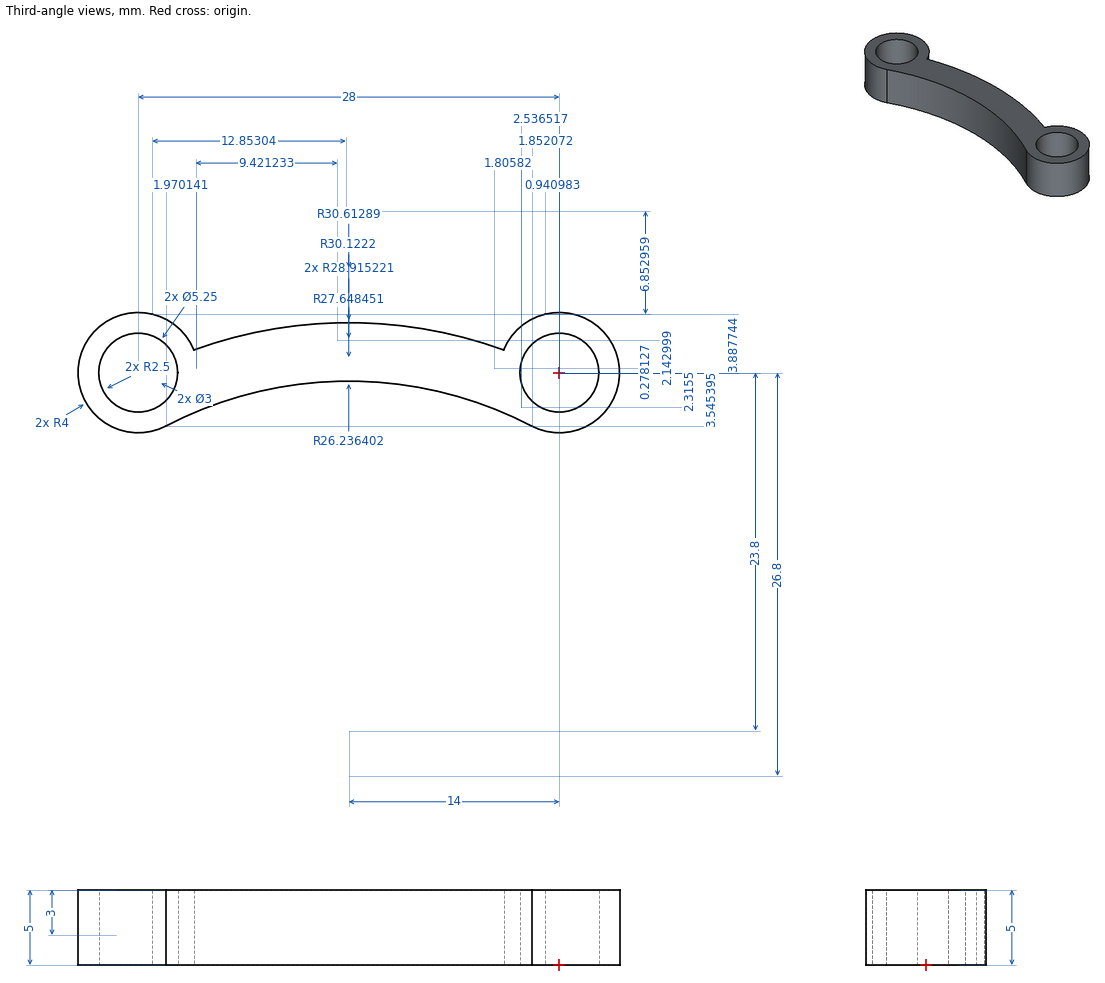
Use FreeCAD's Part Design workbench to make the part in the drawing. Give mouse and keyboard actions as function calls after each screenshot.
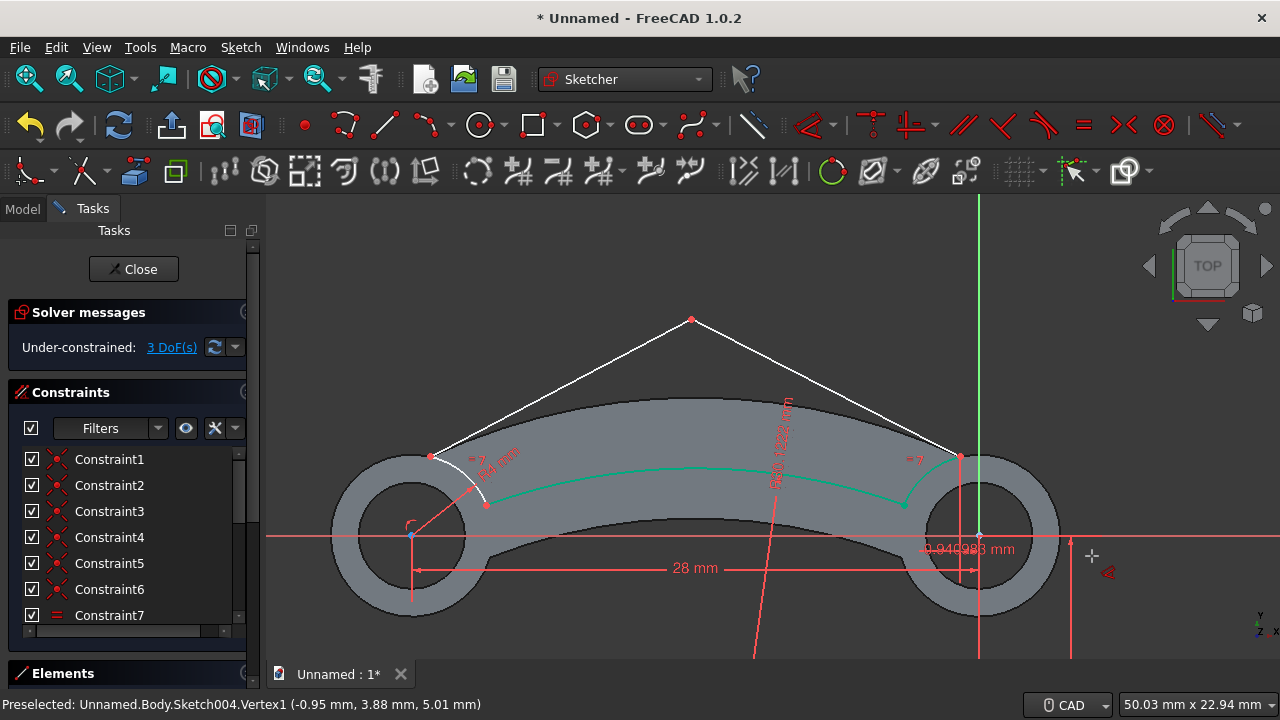
click(431, 457)
click(397, 496)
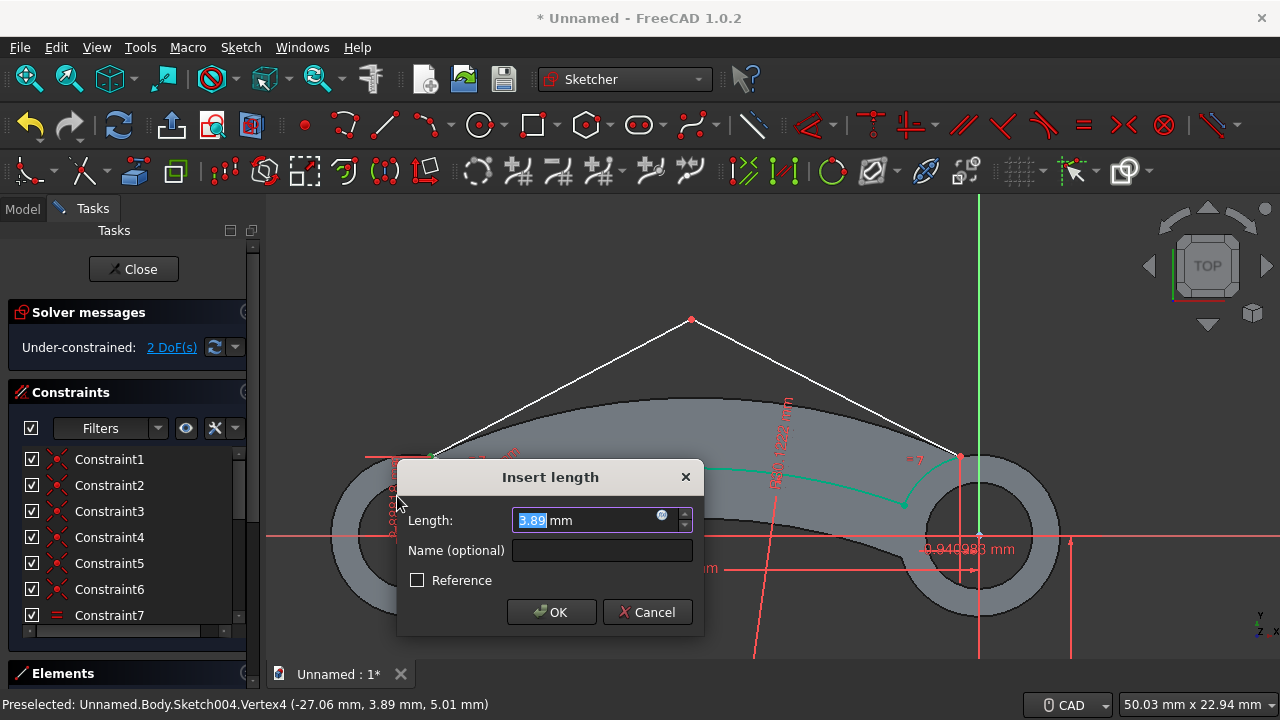
text(3.887744)
key(Return)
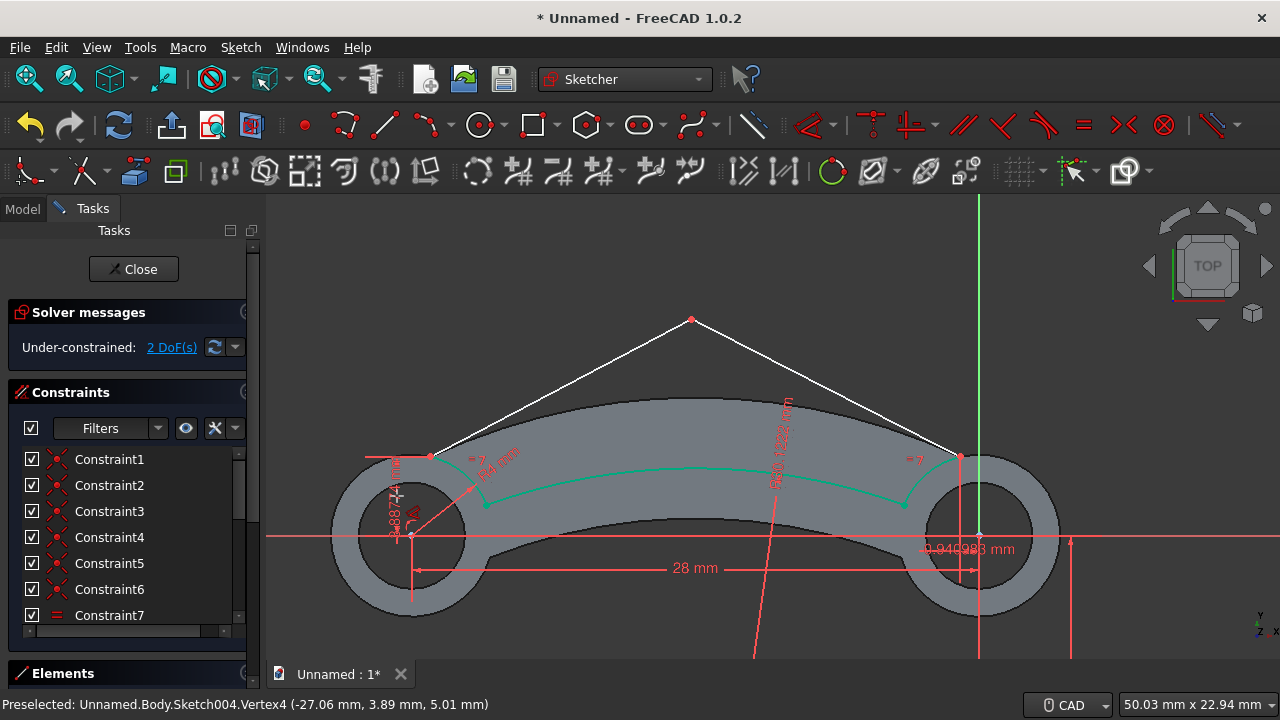
click(880, 416)
click(994, 388)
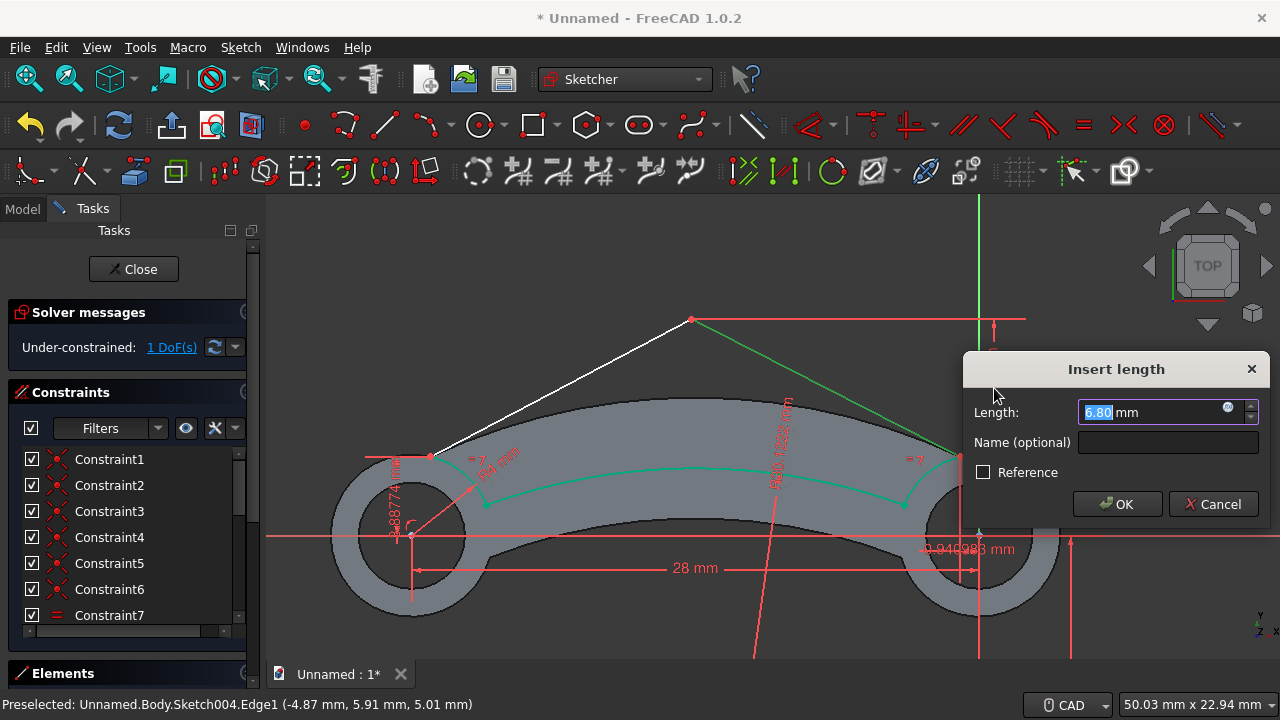
text(6.852959)
key(Return)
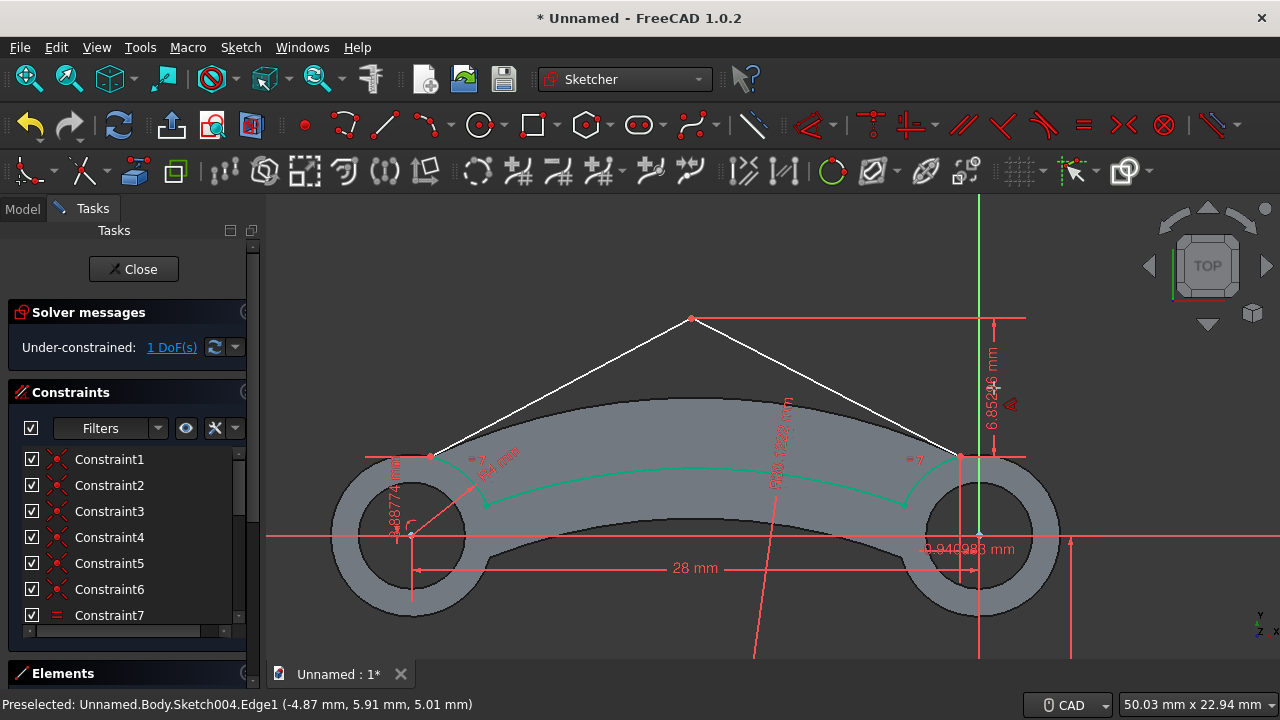
click(614, 360)
click(561, 284)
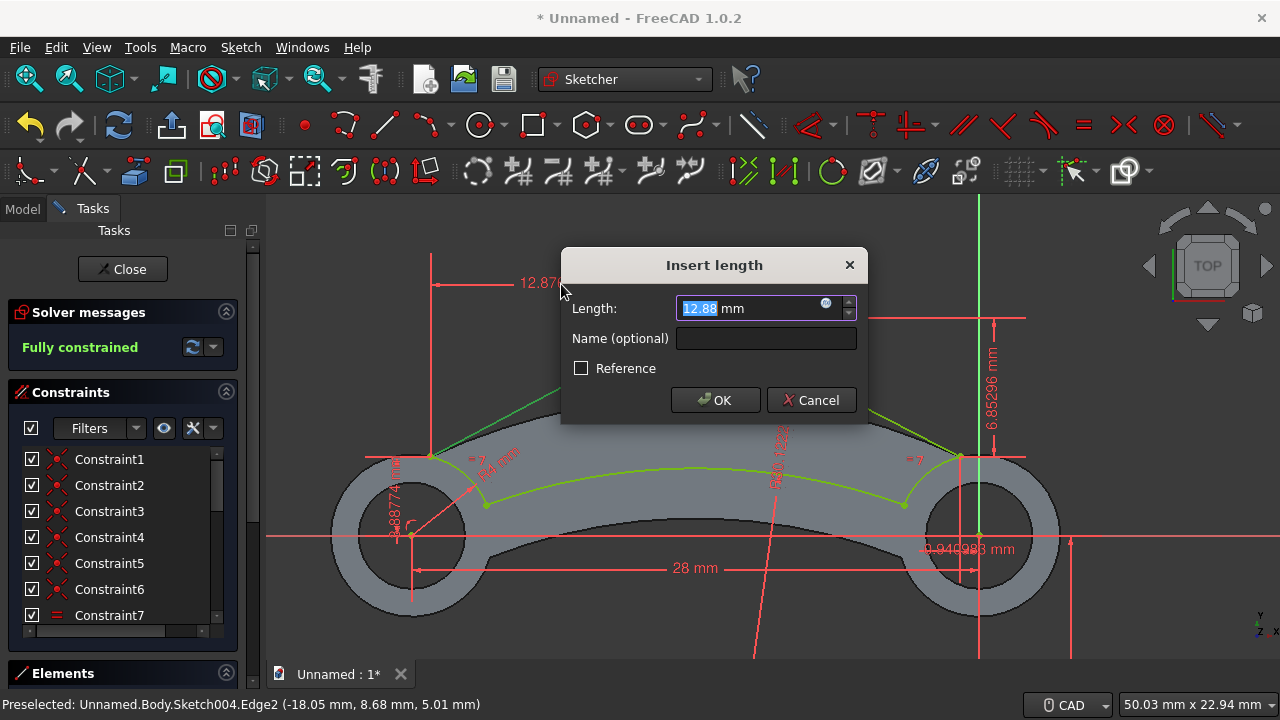
text(12.85304)
key(Return)
key(Escape)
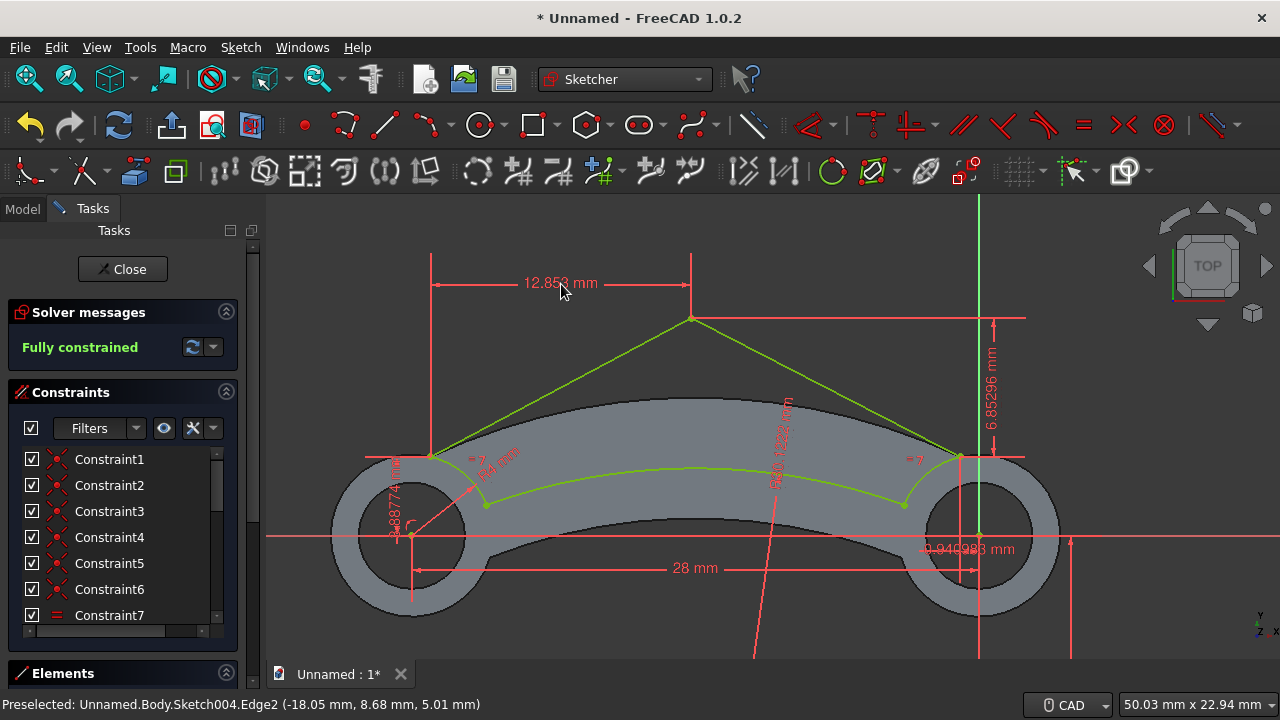
click(123, 269)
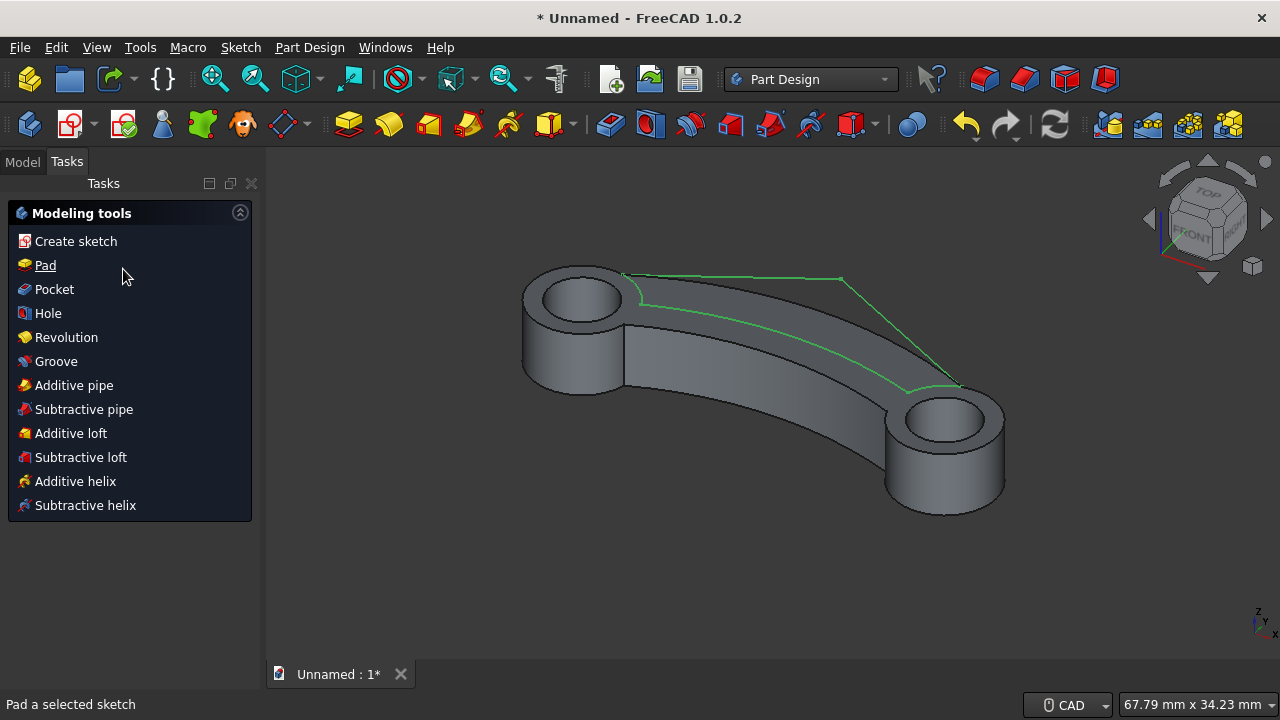
click(612, 124)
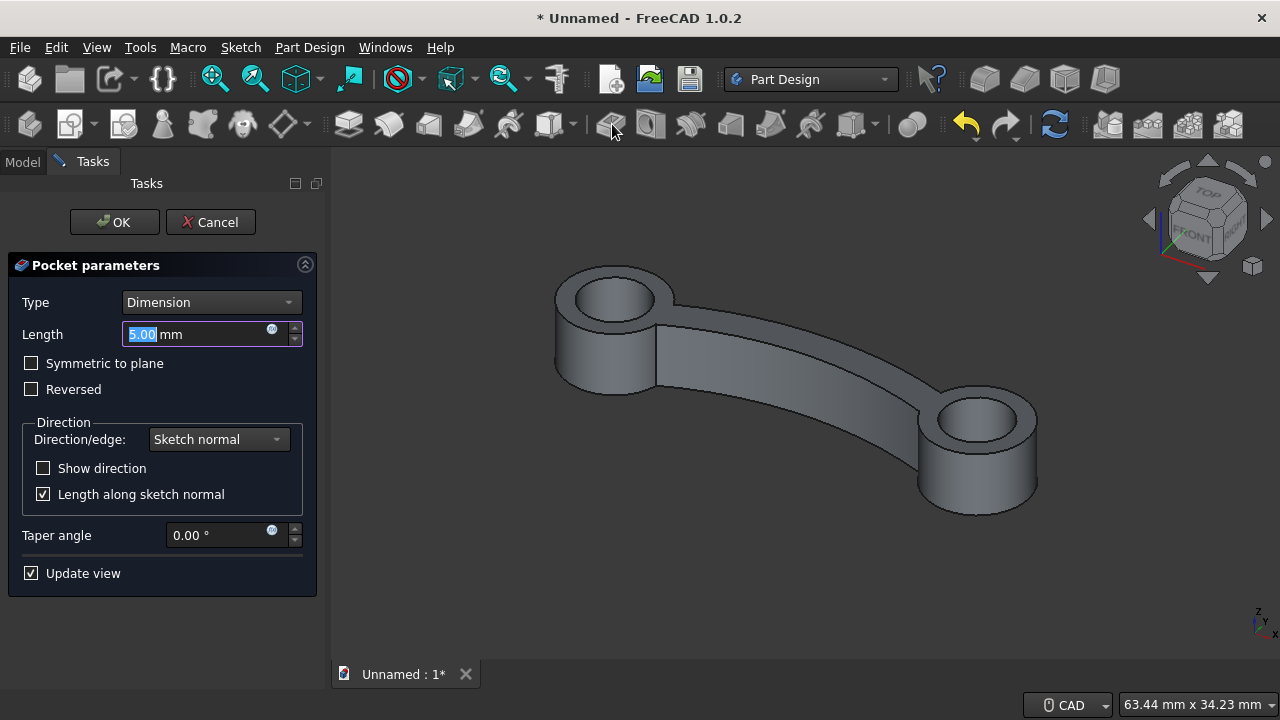
click(212, 302)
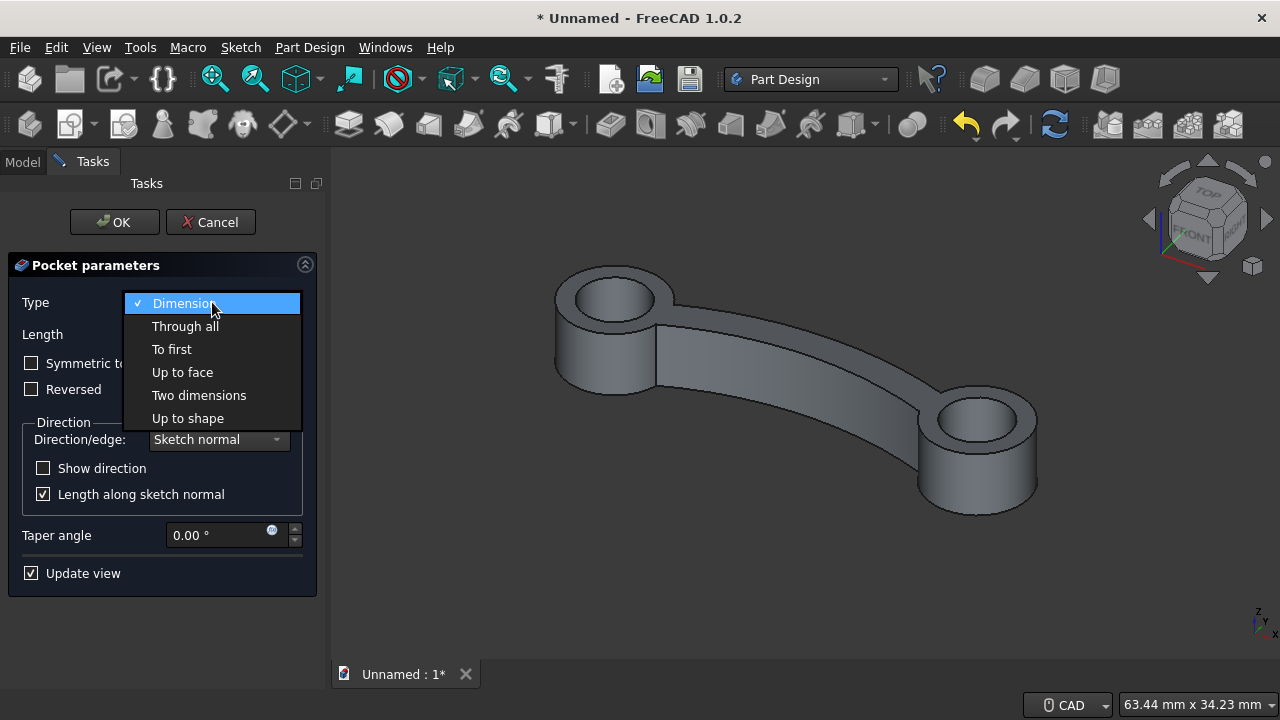
click(212, 326)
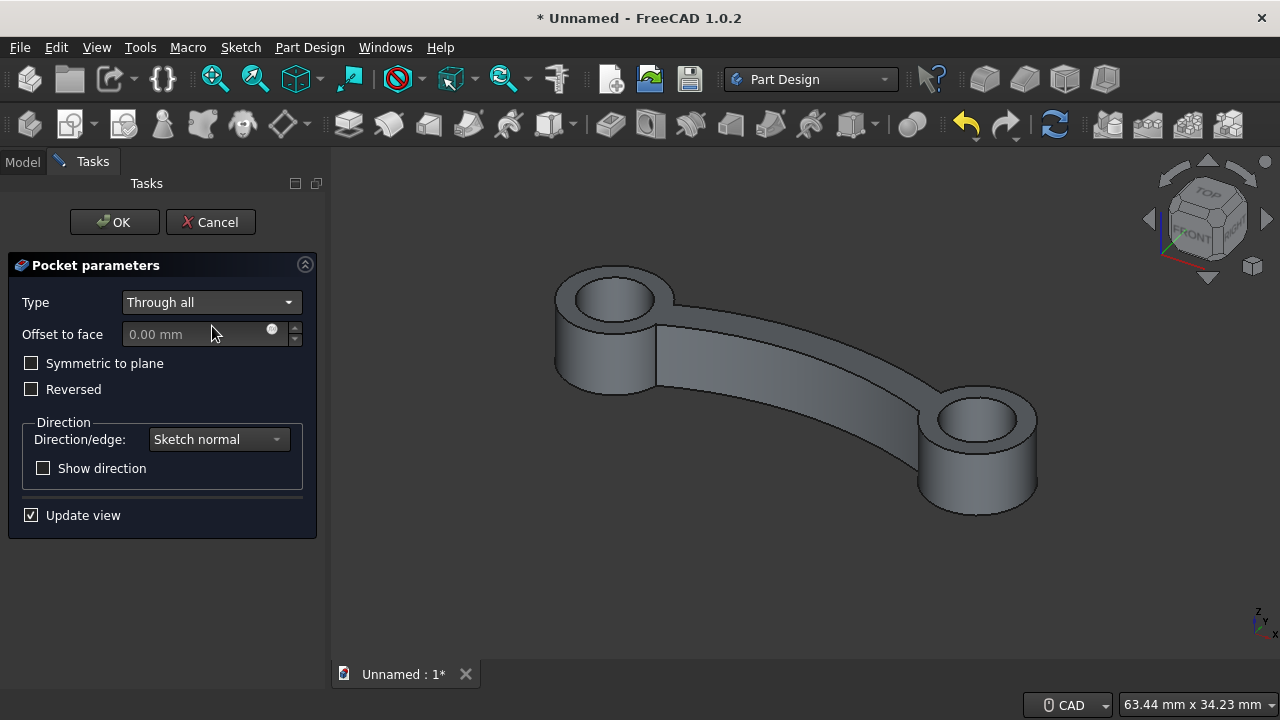
click(115, 222)